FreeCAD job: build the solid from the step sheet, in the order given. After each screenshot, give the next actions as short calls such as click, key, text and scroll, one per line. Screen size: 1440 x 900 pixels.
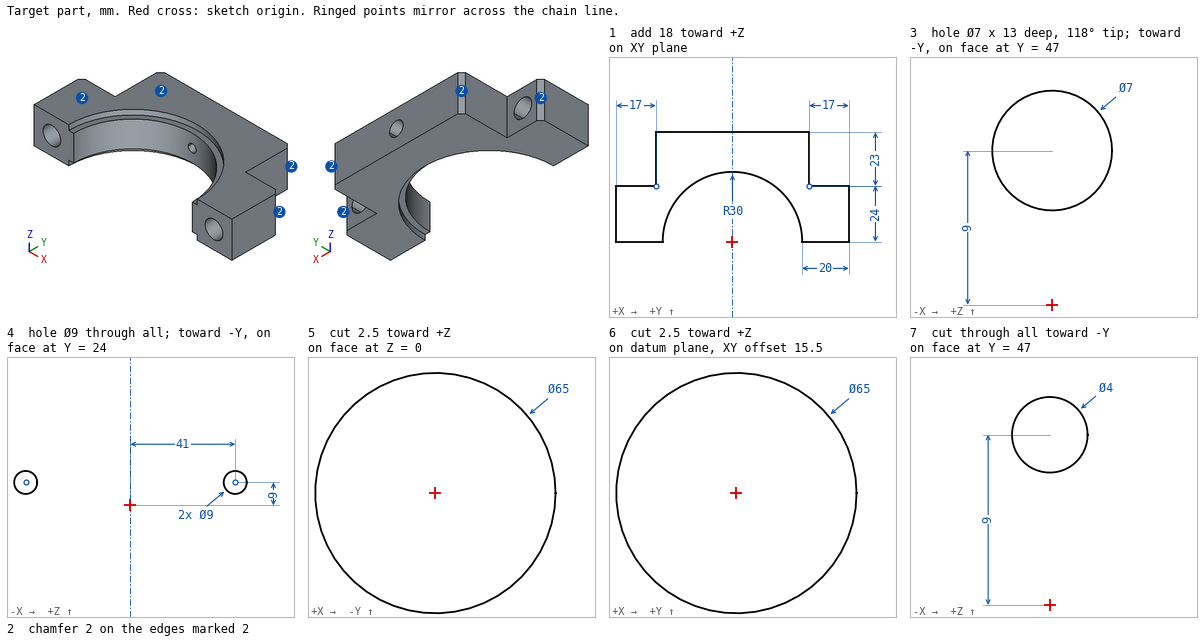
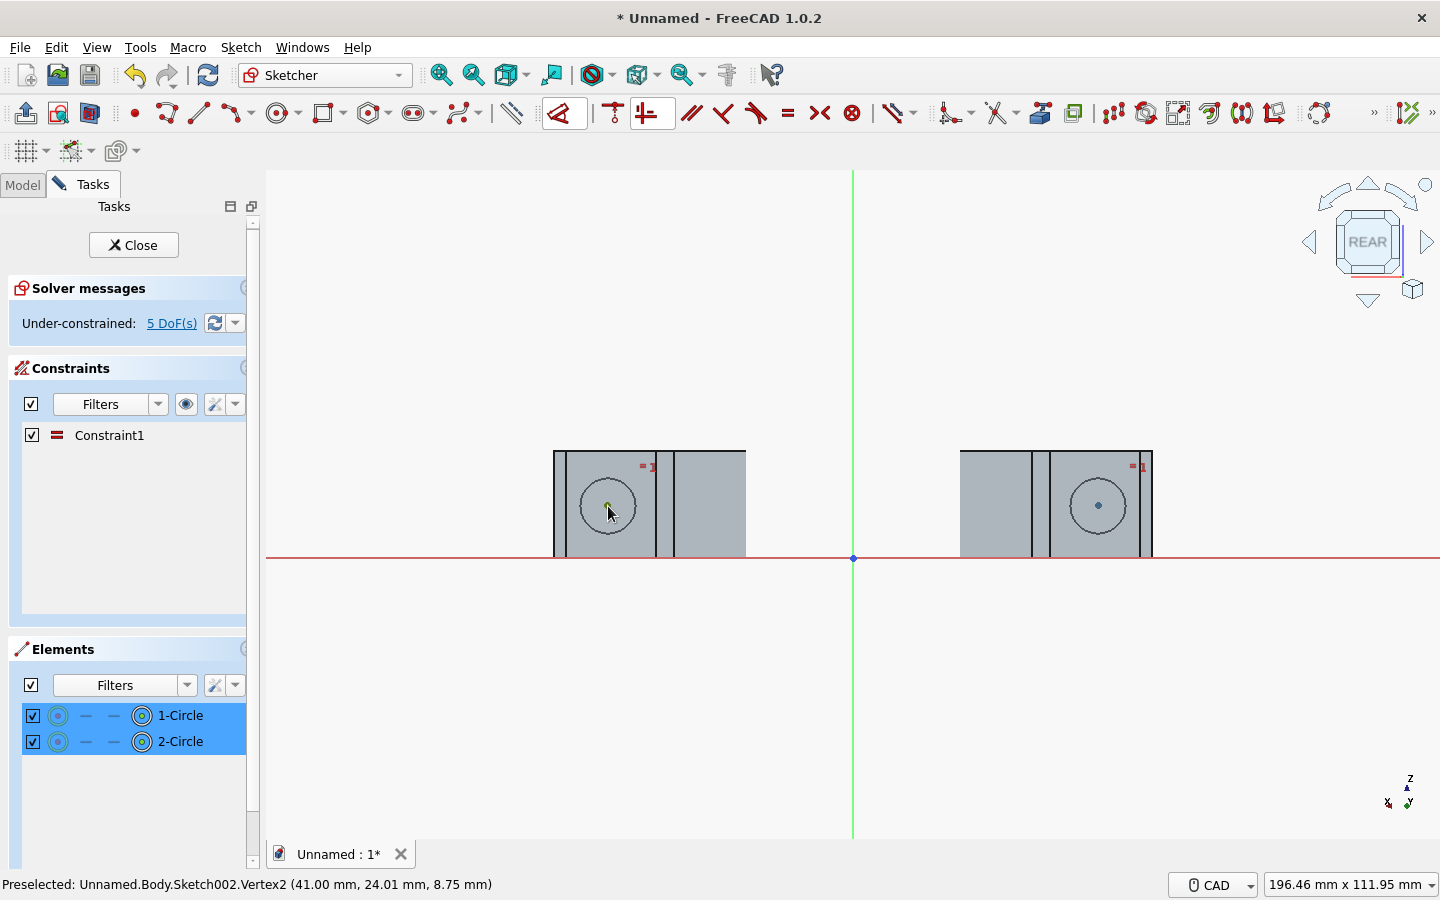
click(853, 767)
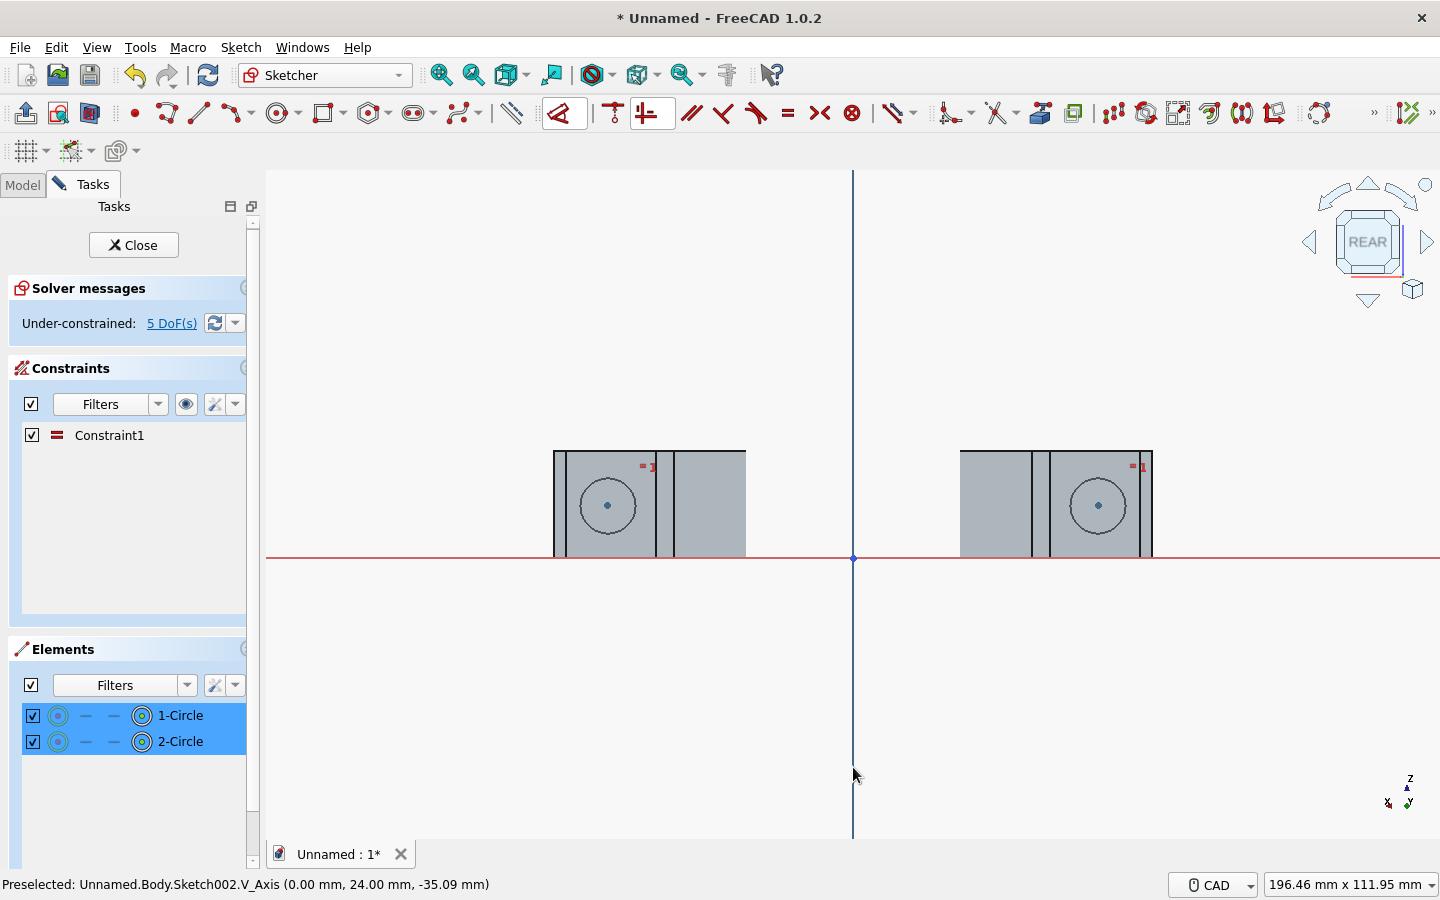
click(820, 114)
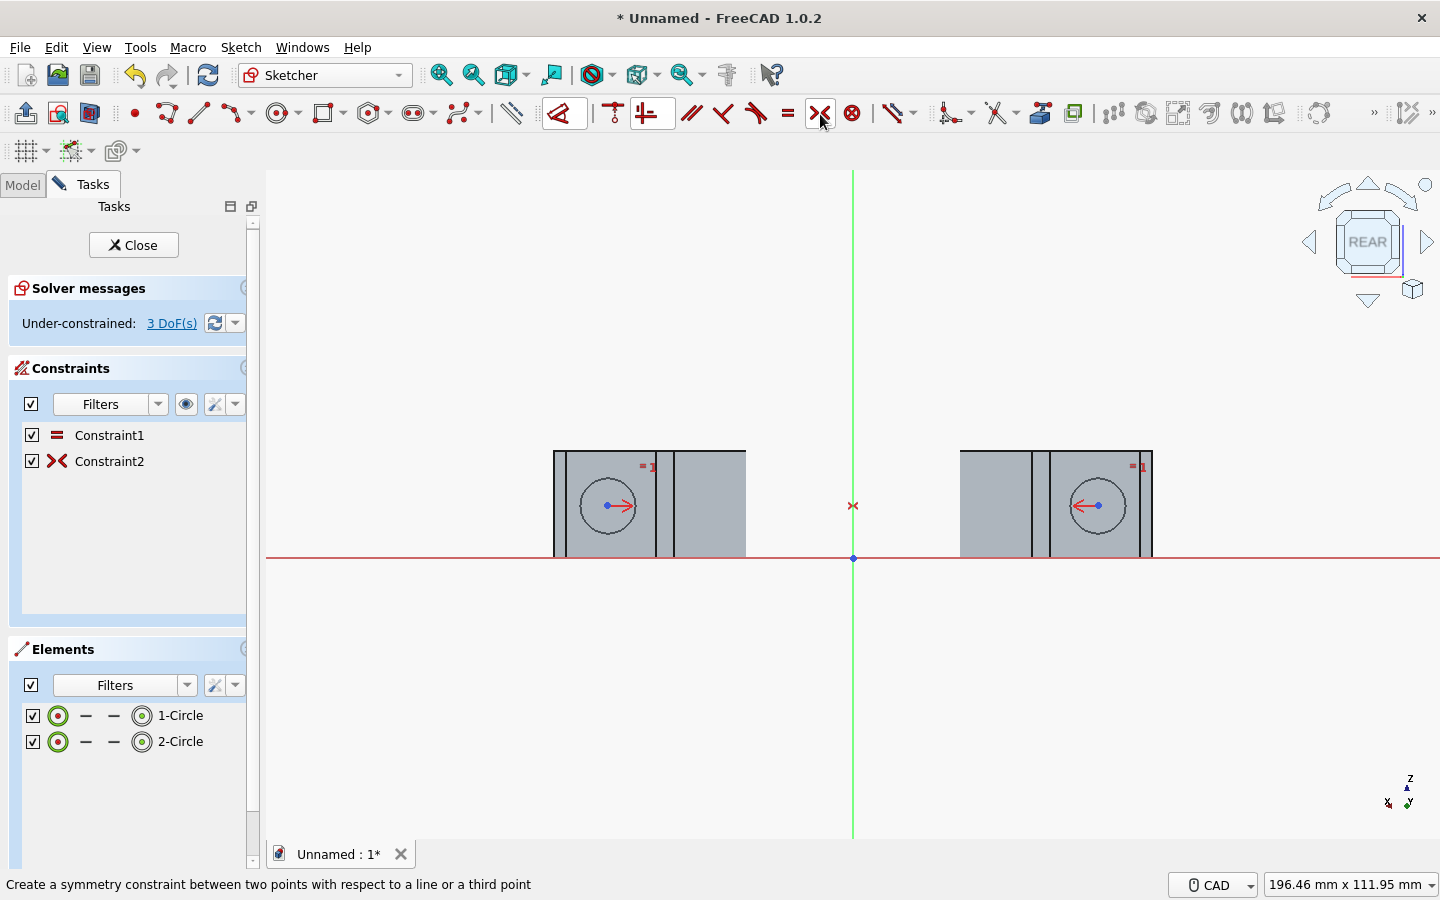
click(1117, 486)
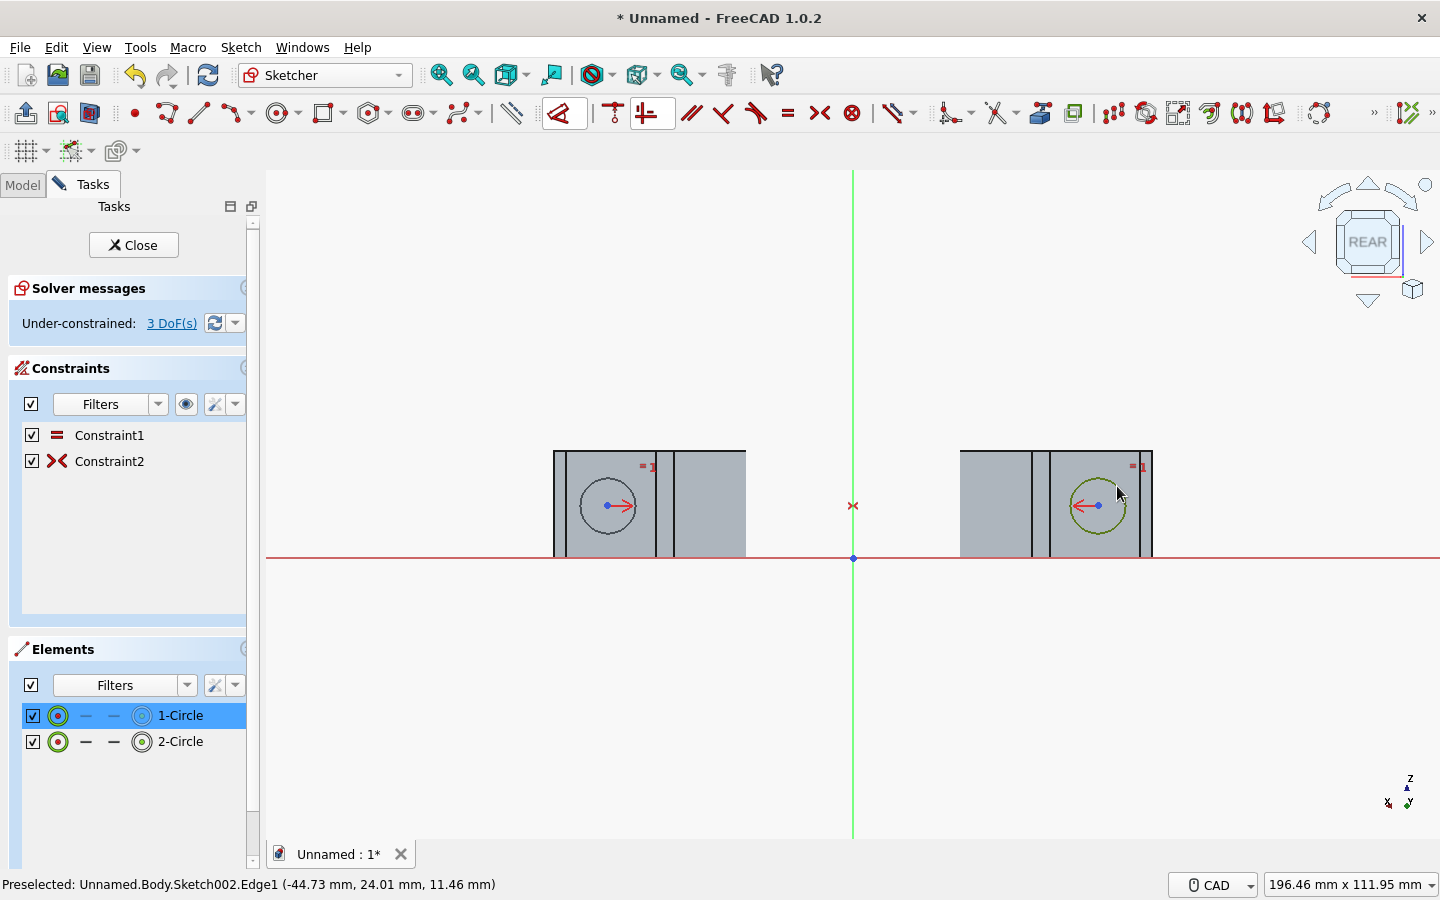
key(k)
key(o)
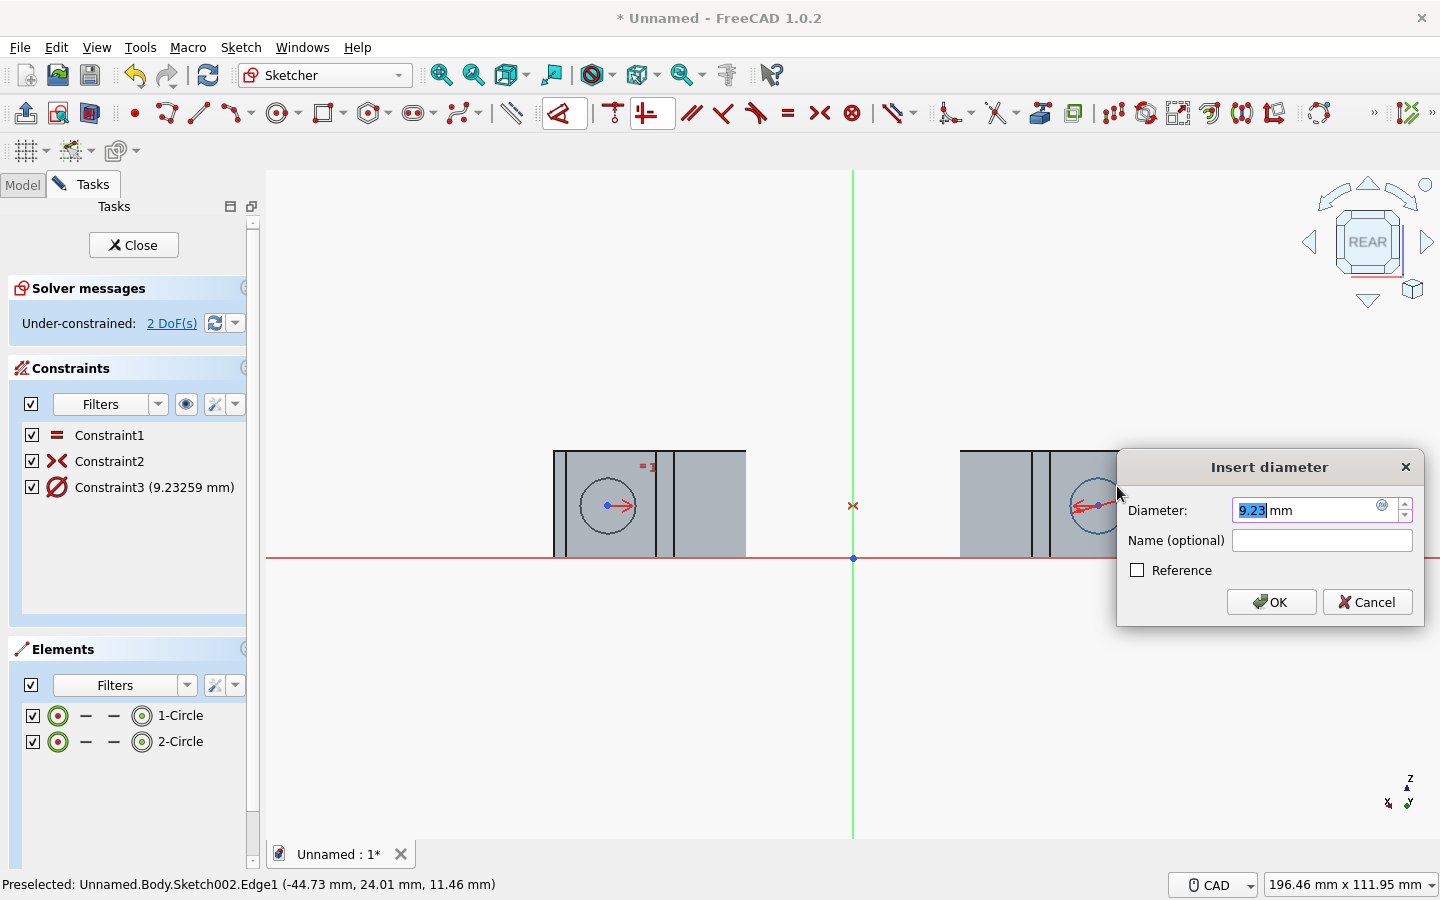
text(9)
key(Return)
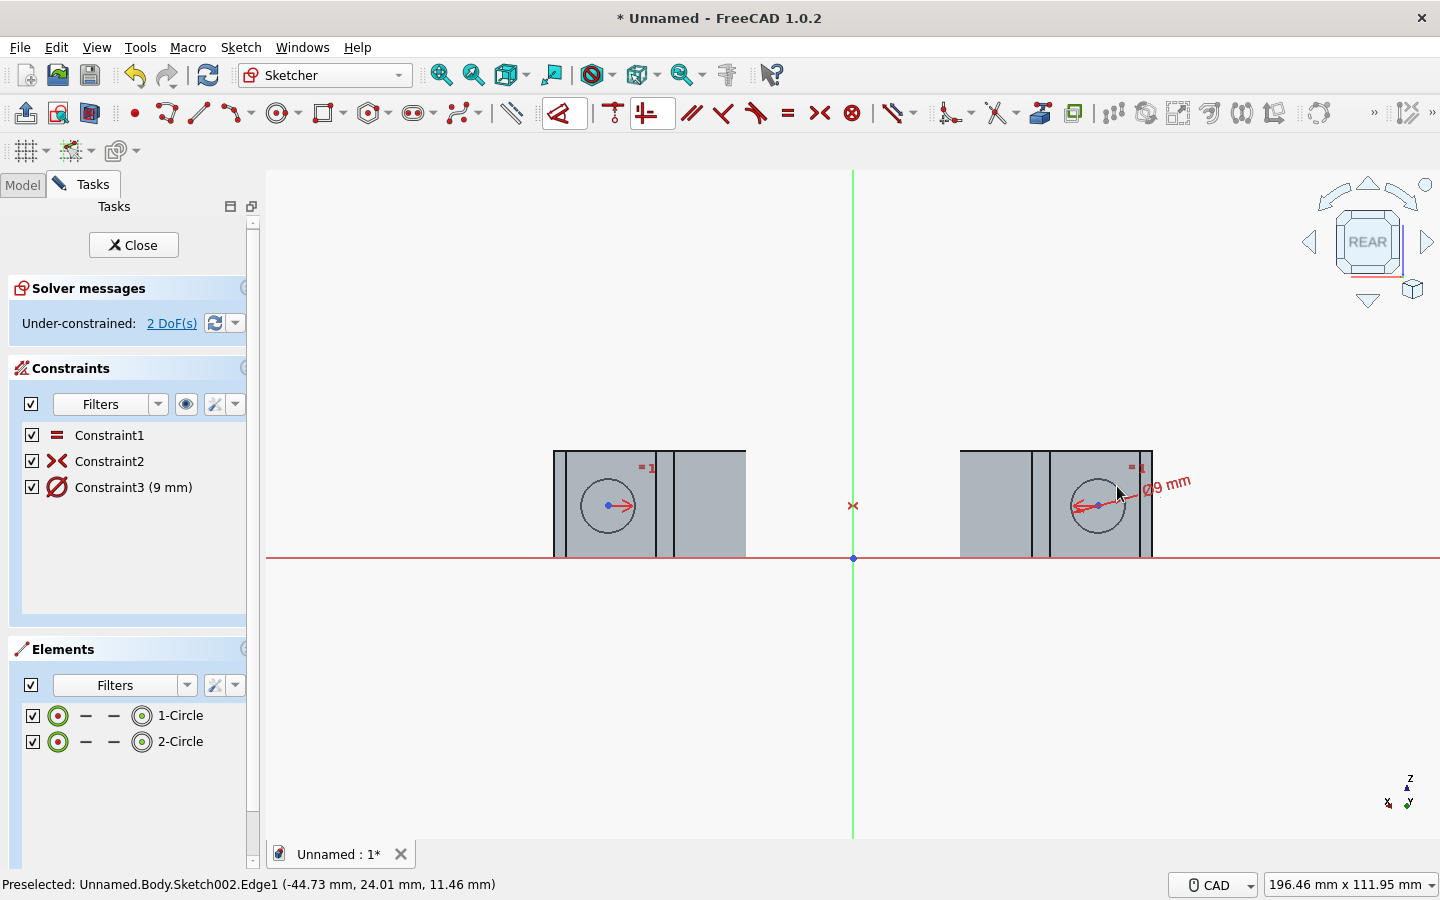
click(1098, 506)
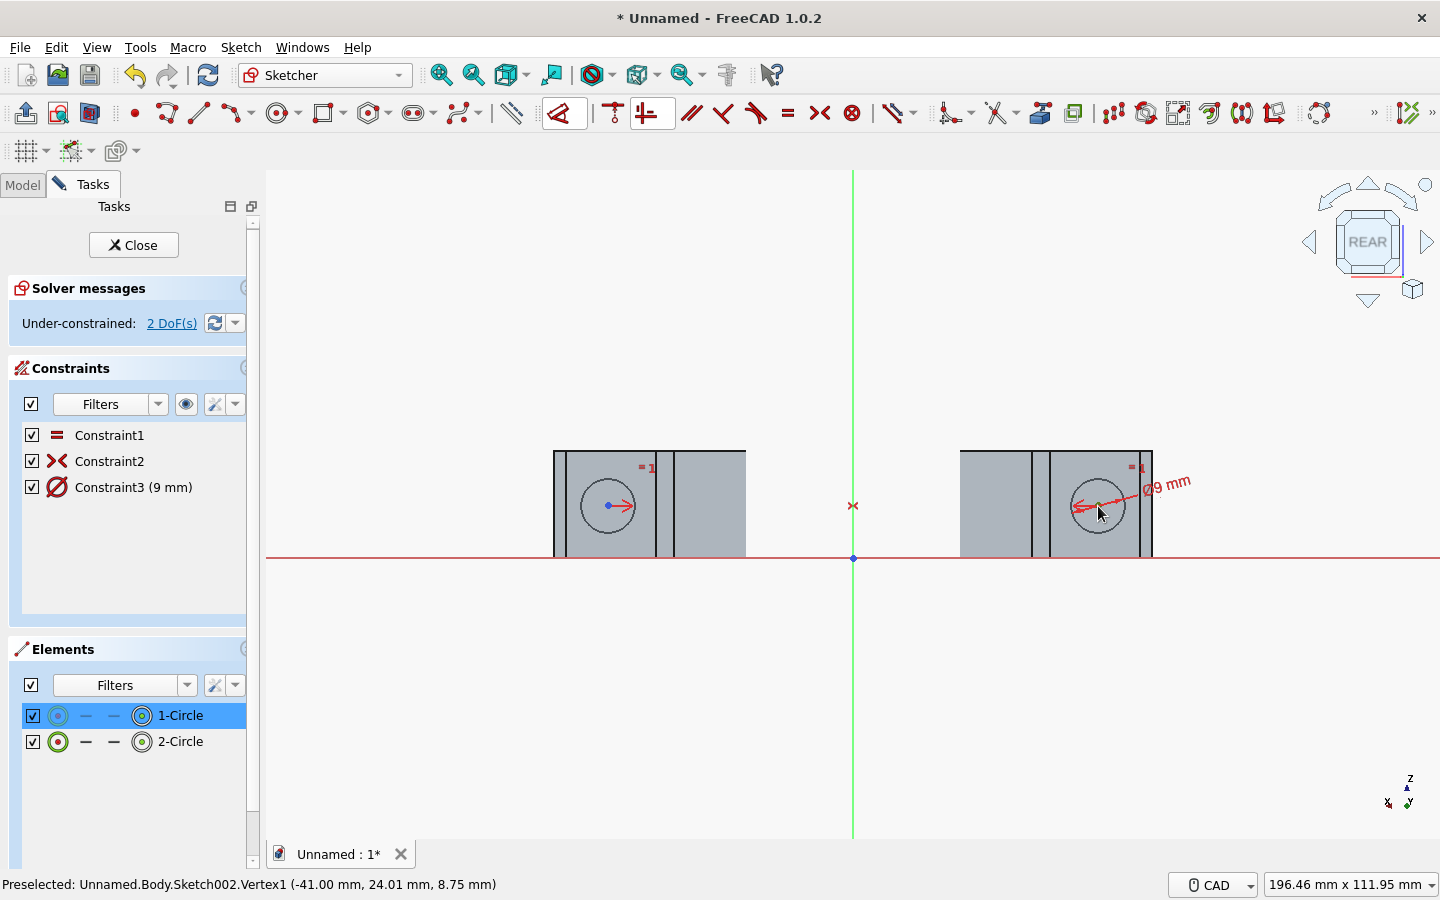
click(582, 114)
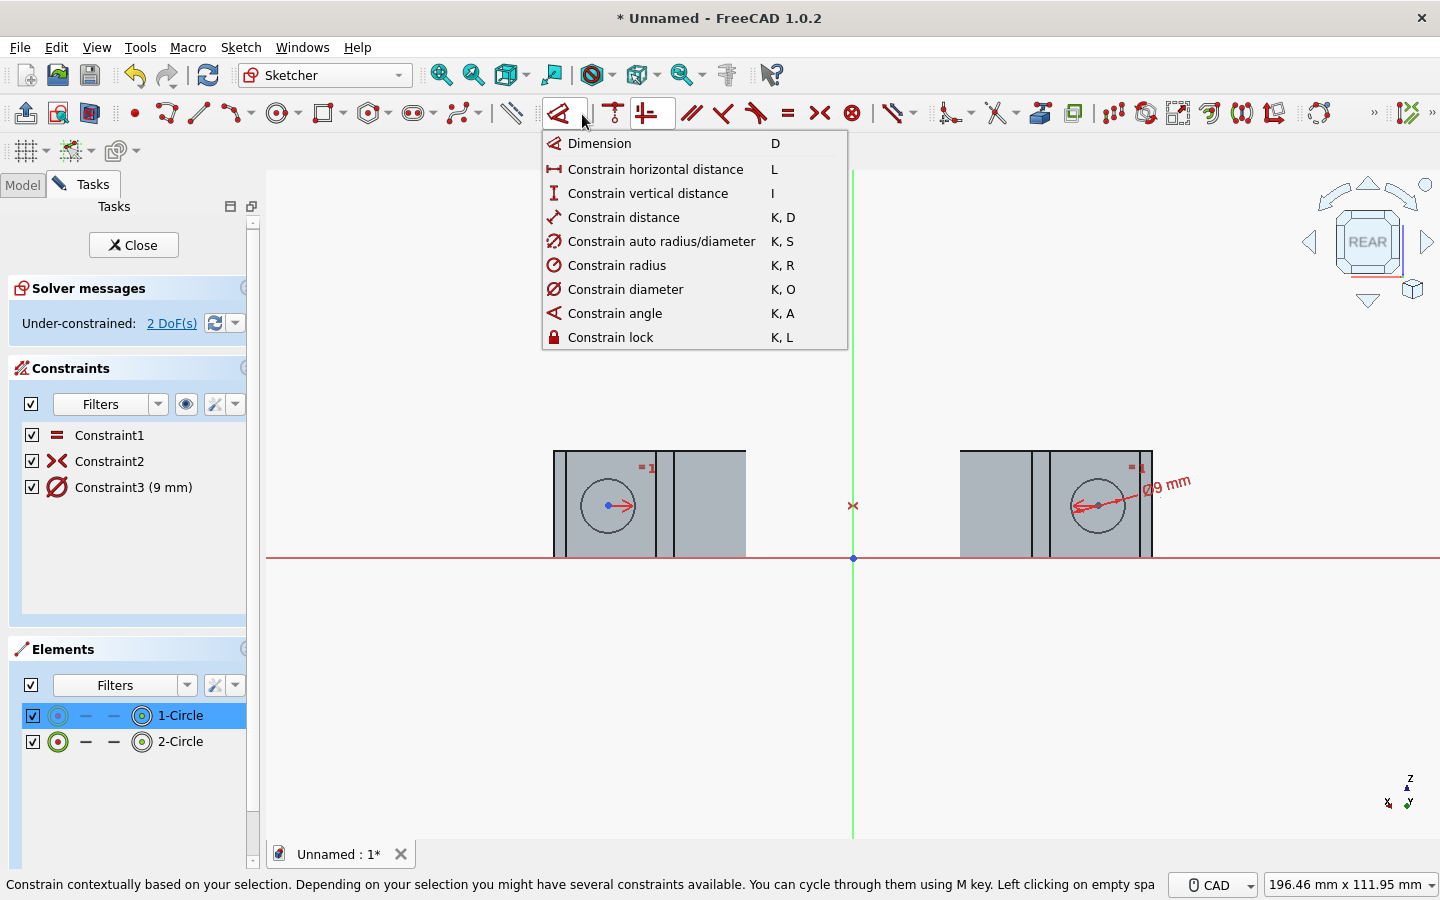
click(695, 193)